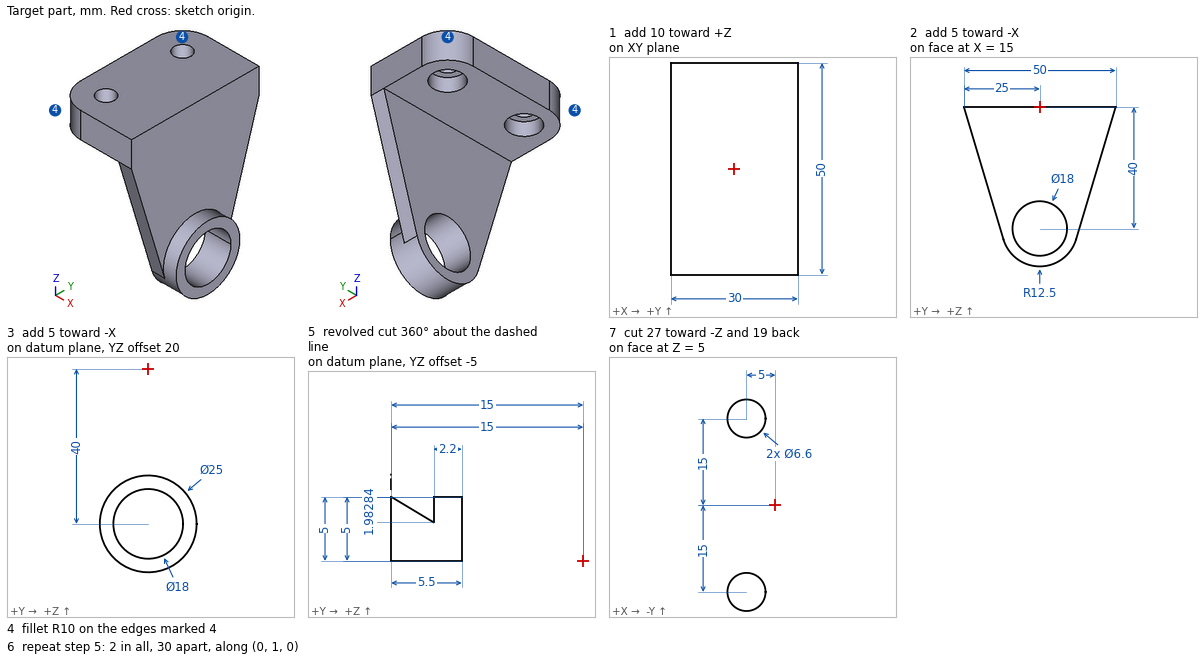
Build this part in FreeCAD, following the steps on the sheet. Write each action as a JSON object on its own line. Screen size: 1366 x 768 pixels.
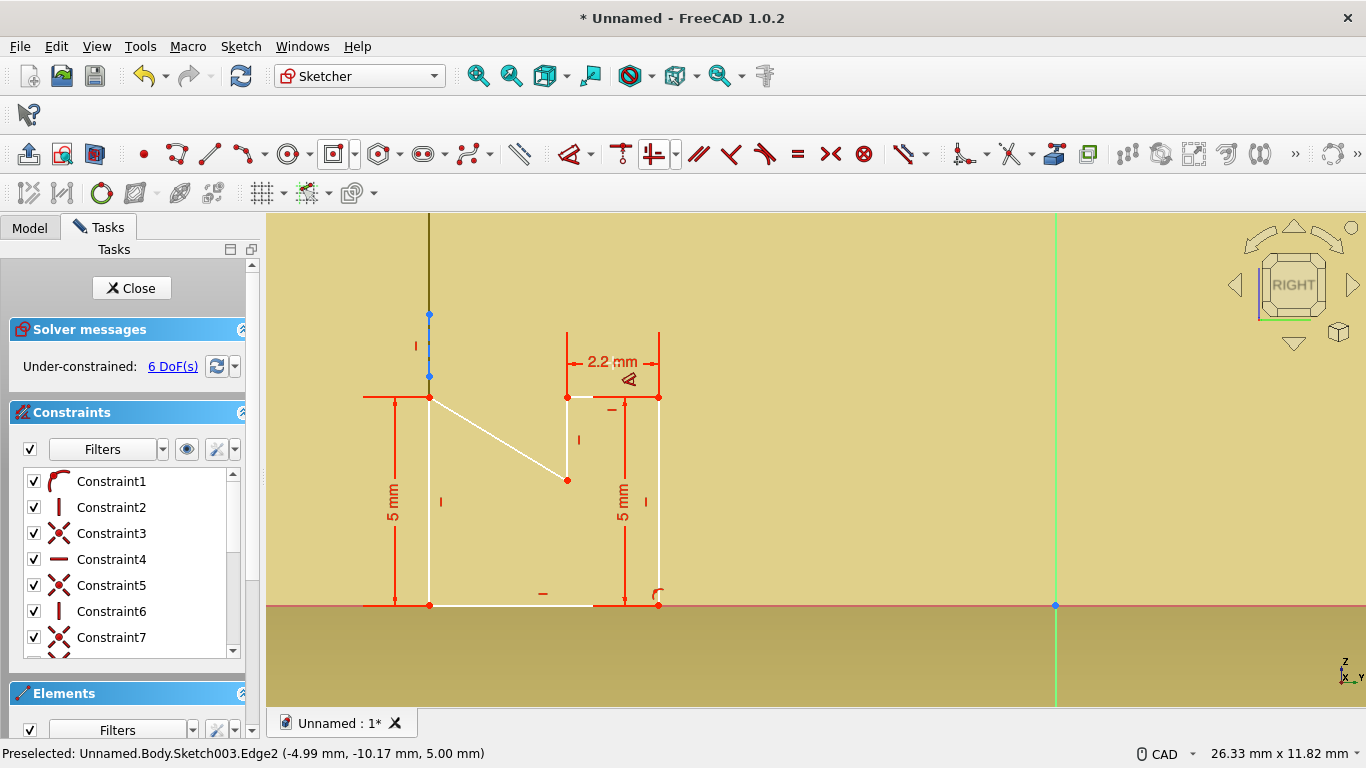
{"action": "left_click", "coordinate": [498, 606]}
{"action": "left_click", "coordinate": [544, 640]}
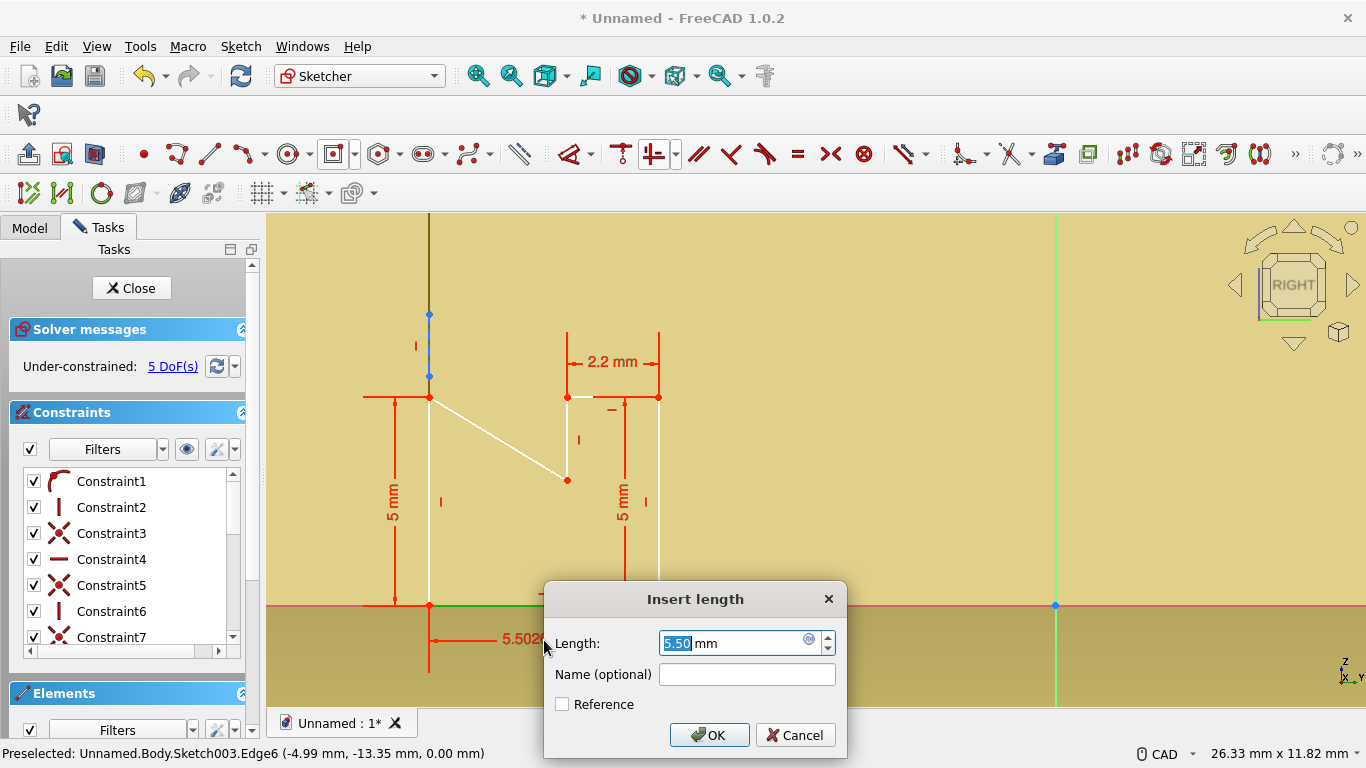
{"action": "type", "text": "5.5"}
{"action": "key", "text": "Return"}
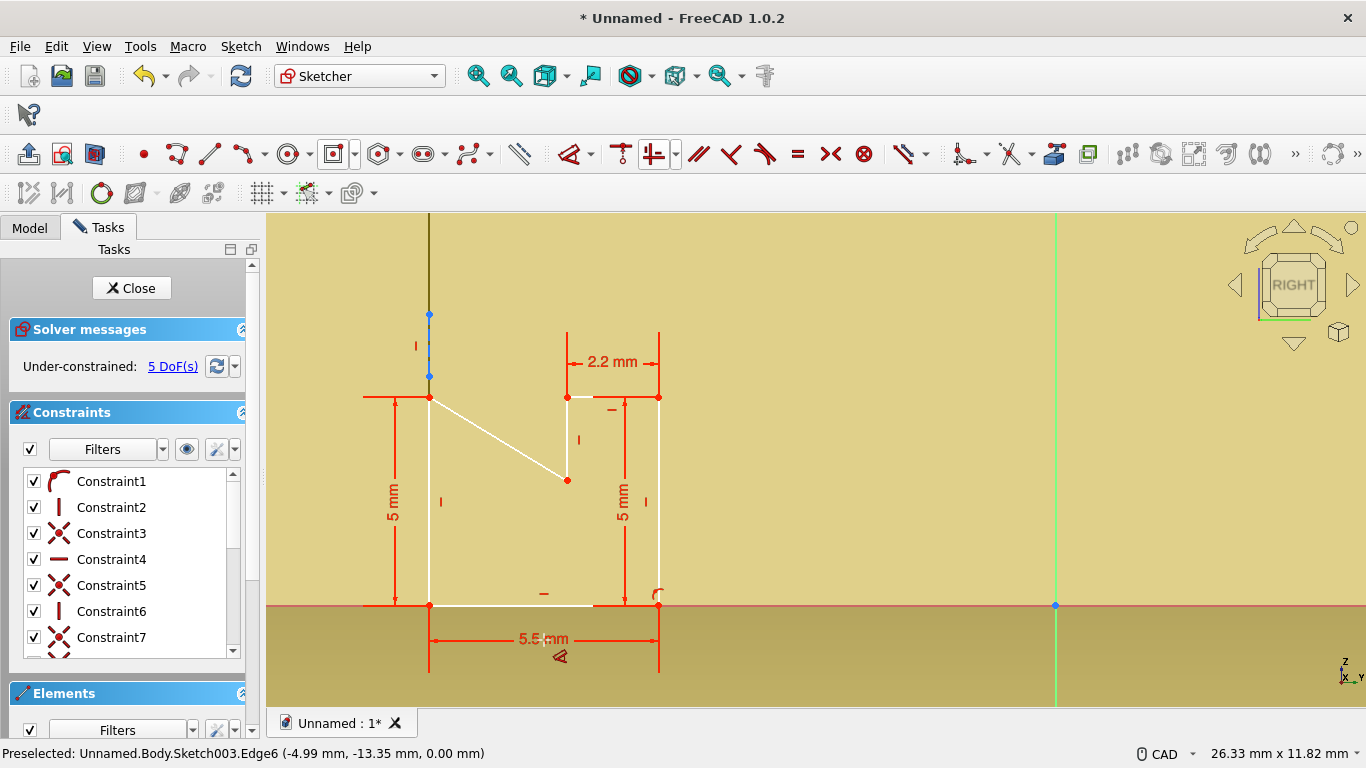
{"action": "left_click", "coordinate": [429, 397]}
{"action": "left_click", "coordinate": [742, 640]}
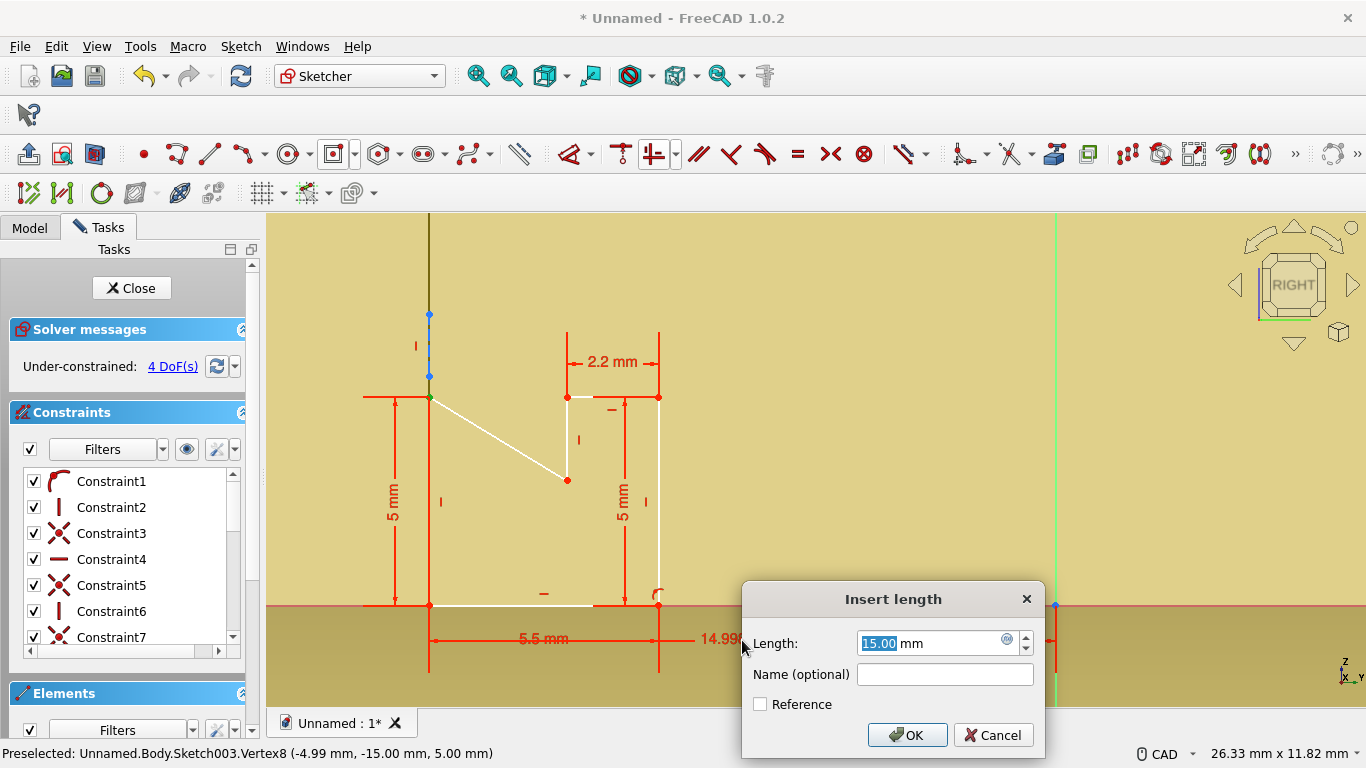
{"action": "type", "text": "15"}
{"action": "key", "text": "Return"}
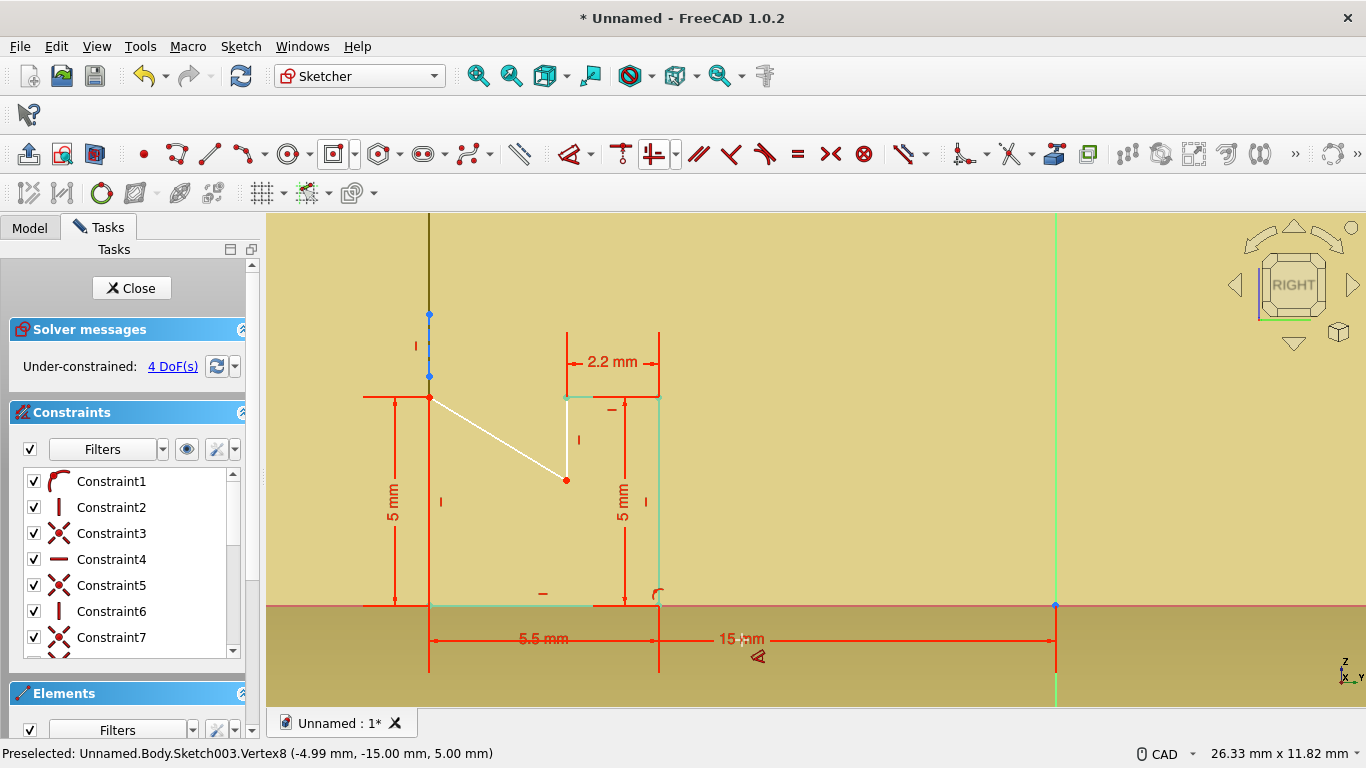
{"action": "left_click", "coordinate": [429, 377]}
{"action": "left_click", "coordinate": [887, 640]}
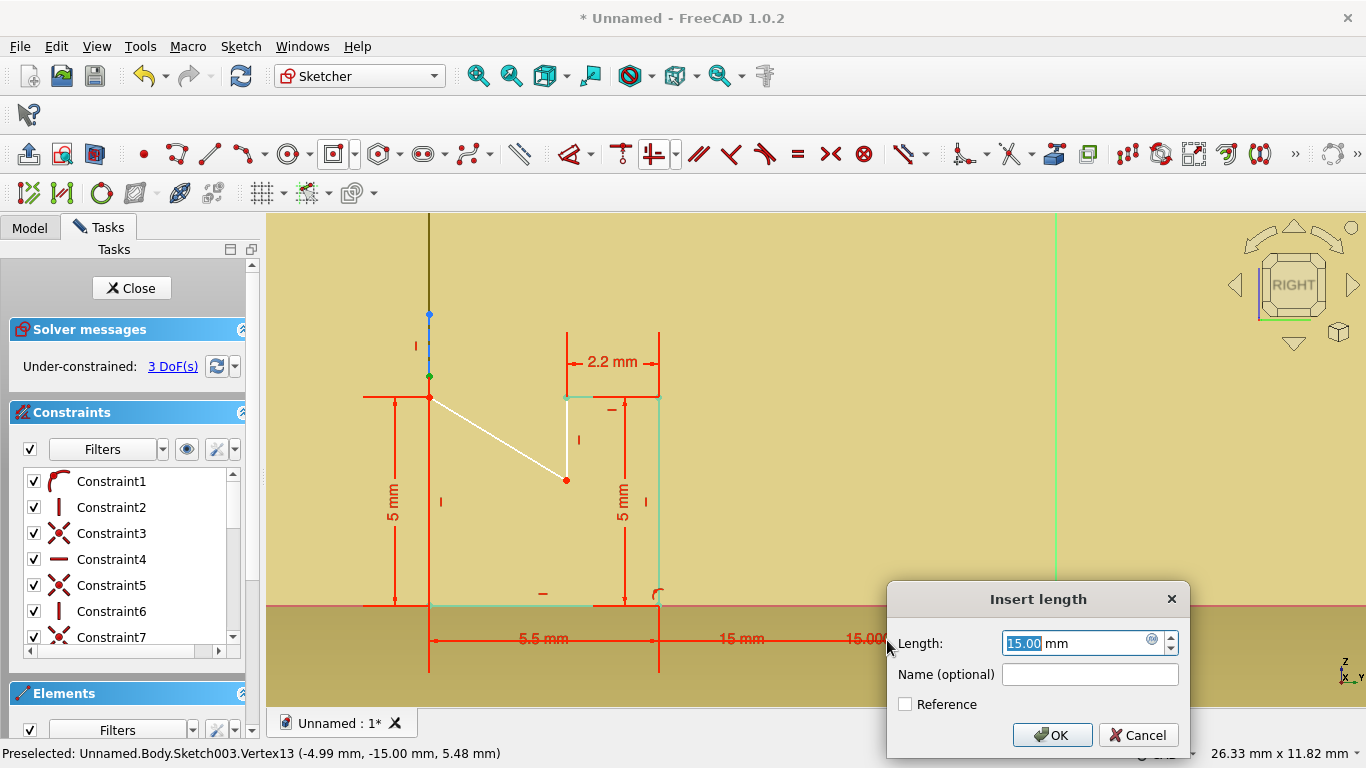
{"action": "type", "text": "15"}
{"action": "key", "text": "Return"}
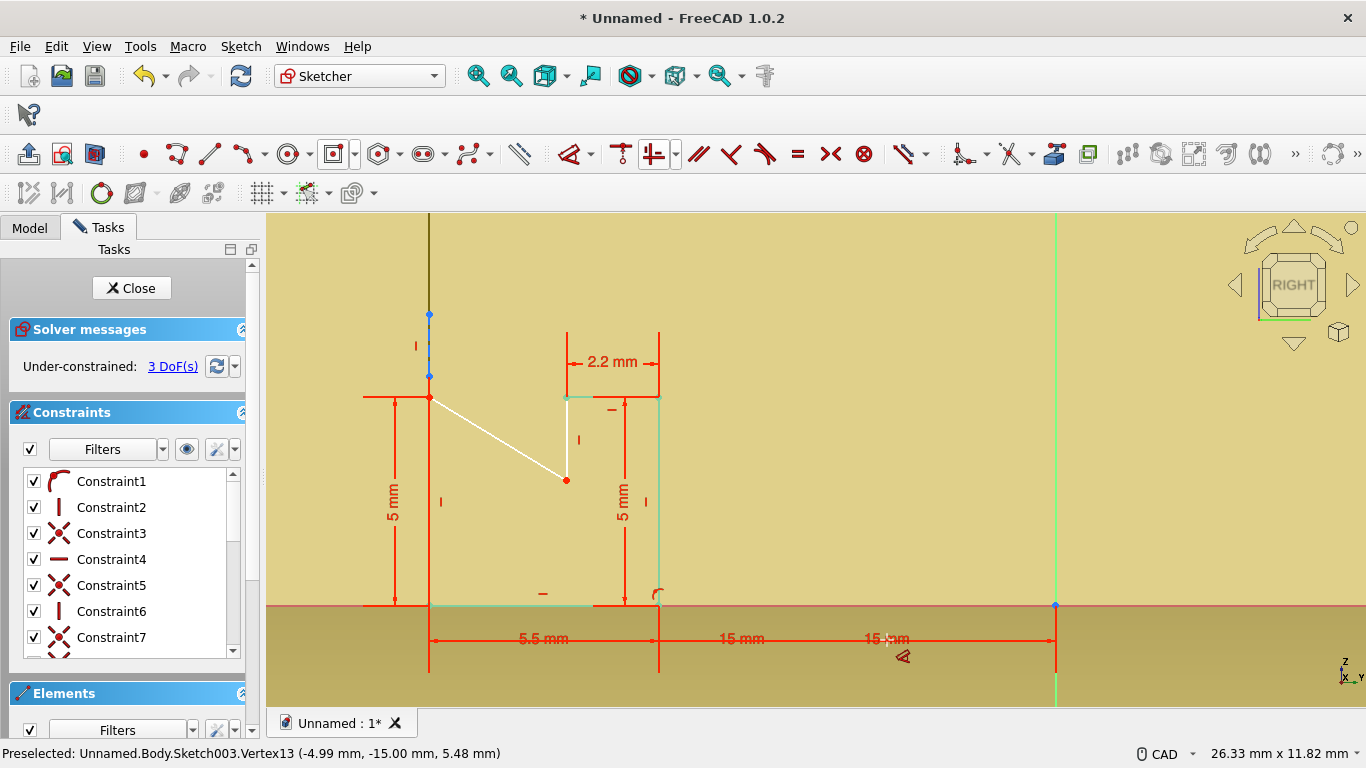
{"action": "left_click", "coordinate": [567, 422]}
{"action": "left_click", "coordinate": [533, 439]}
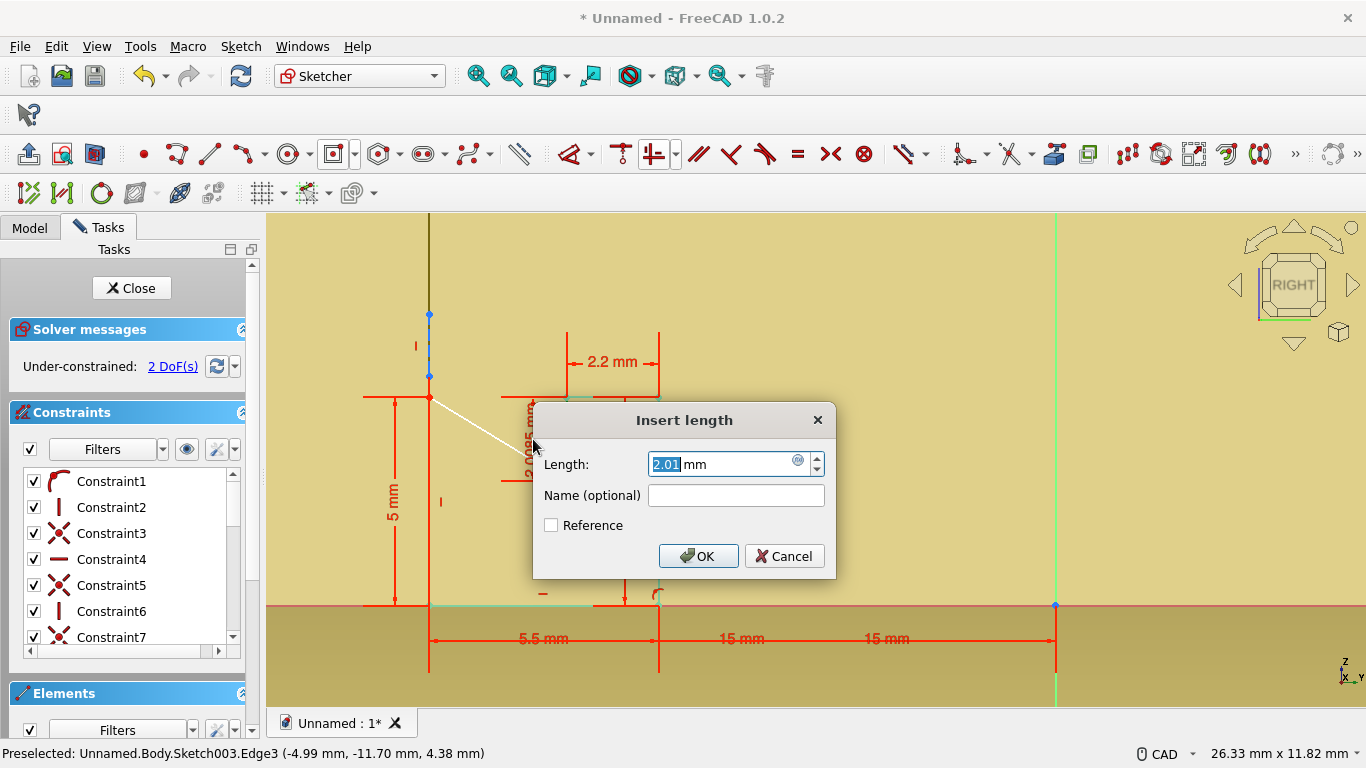
{"action": "type", "text": "1.98284"}
{"action": "key", "text": "Return"}
{"action": "key", "text": "Escape"}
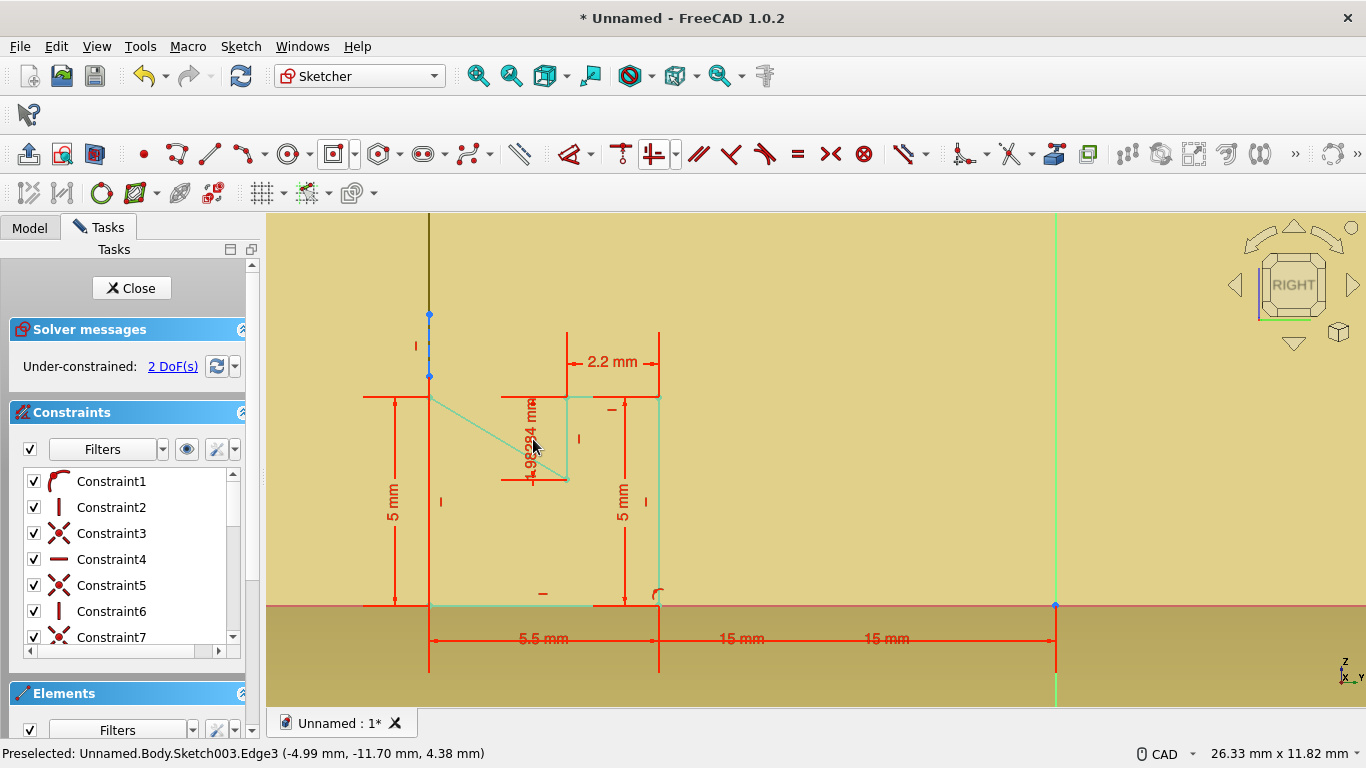
{"action": "left_click", "coordinate": [132, 288]}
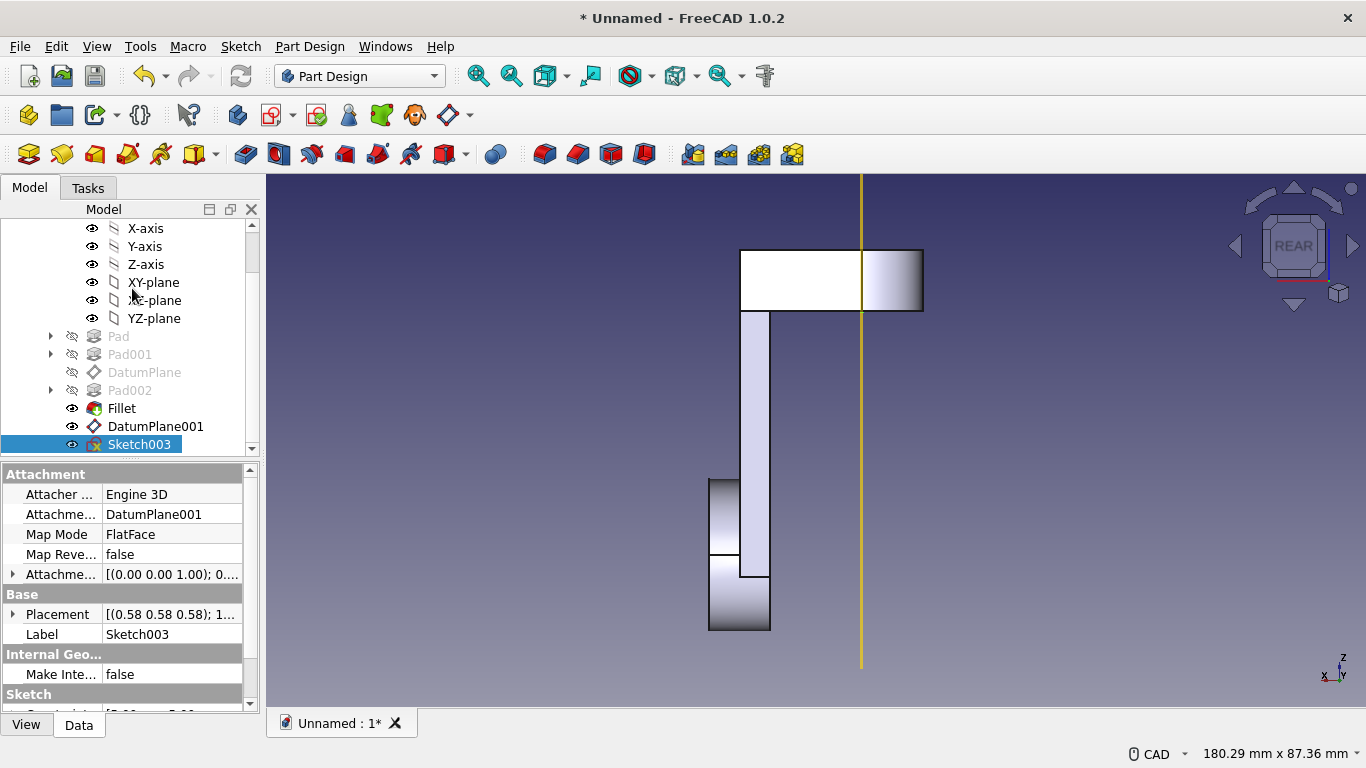
{"action": "left_click", "coordinate": [312, 154]}